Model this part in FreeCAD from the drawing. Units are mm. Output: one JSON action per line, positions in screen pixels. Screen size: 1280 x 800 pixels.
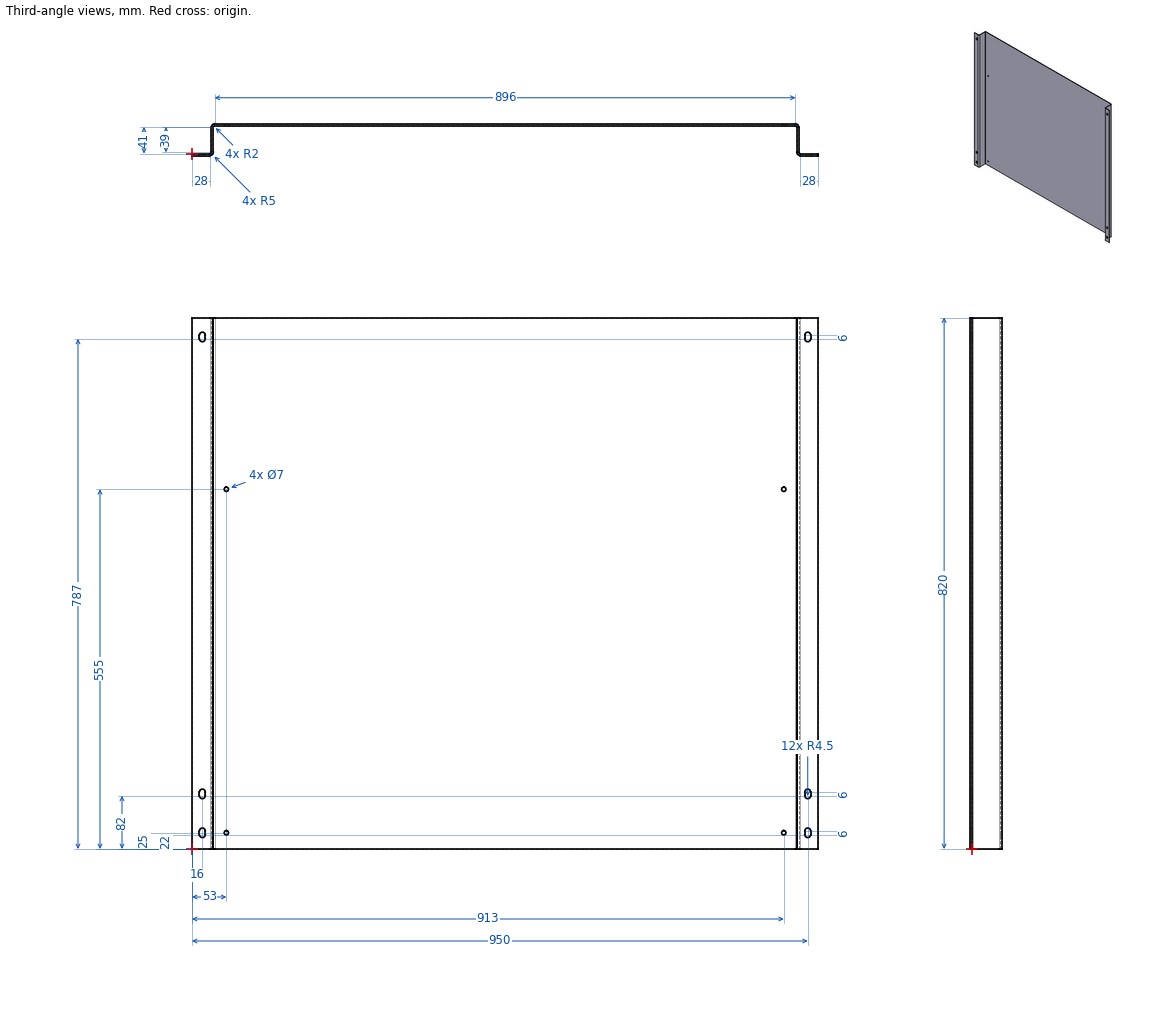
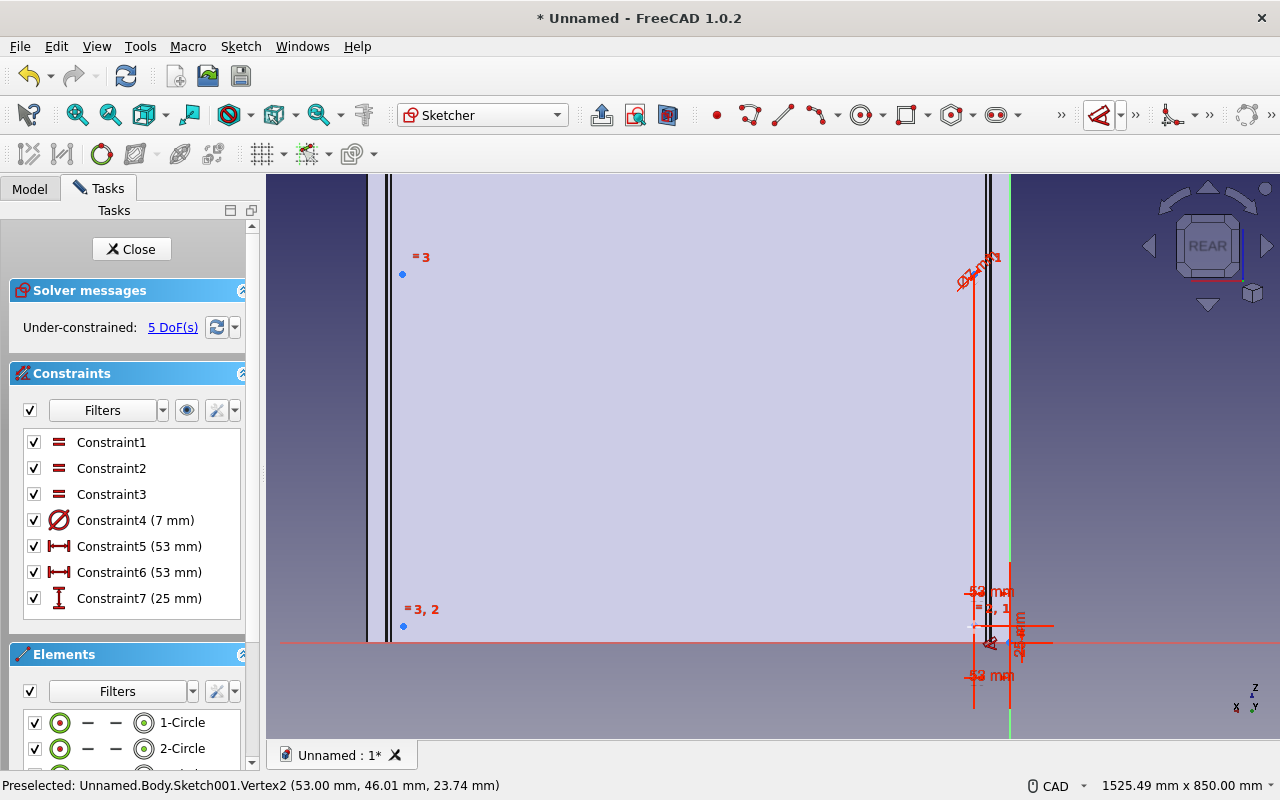
{"action": "scroll", "coordinate": [403, 627], "scroll_direction": "up", "scroll_amount": 5}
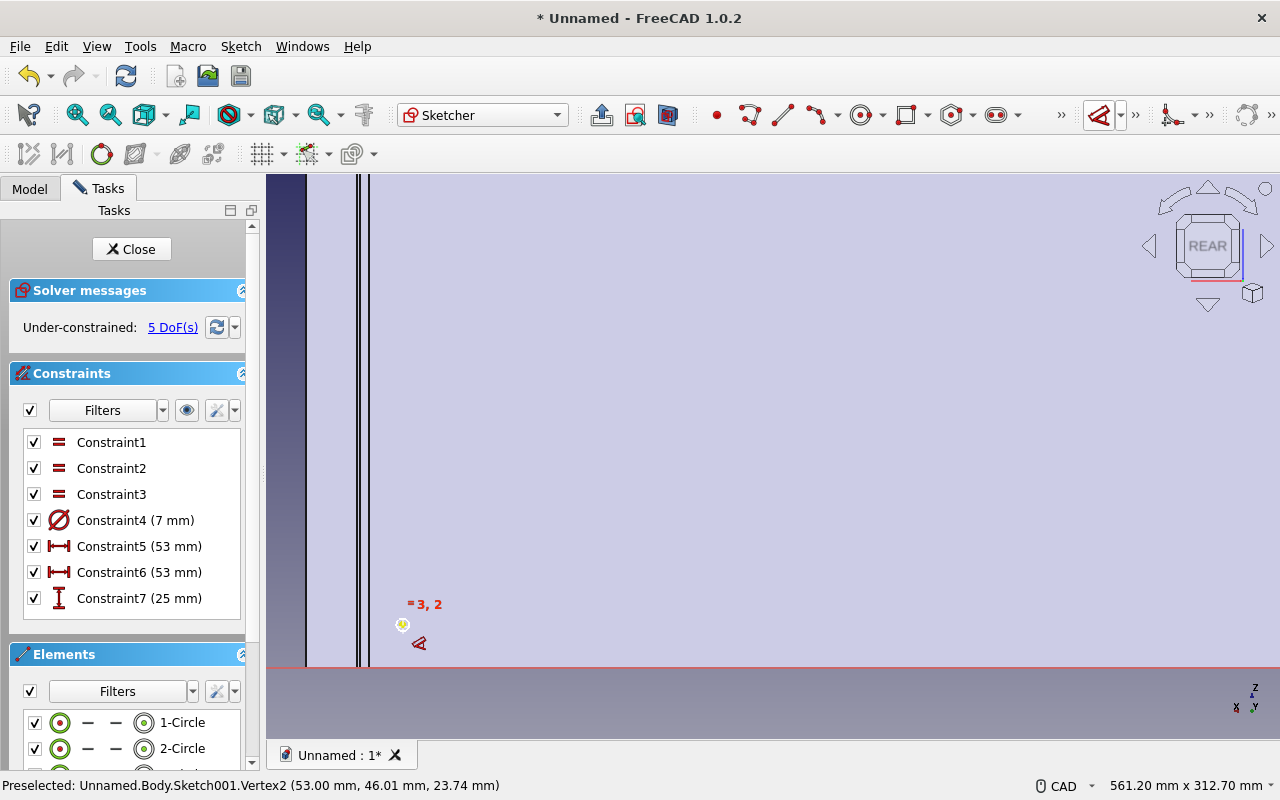
{"action": "left_click", "coordinate": [403, 625]}
{"action": "left_click", "coordinate": [369, 646]}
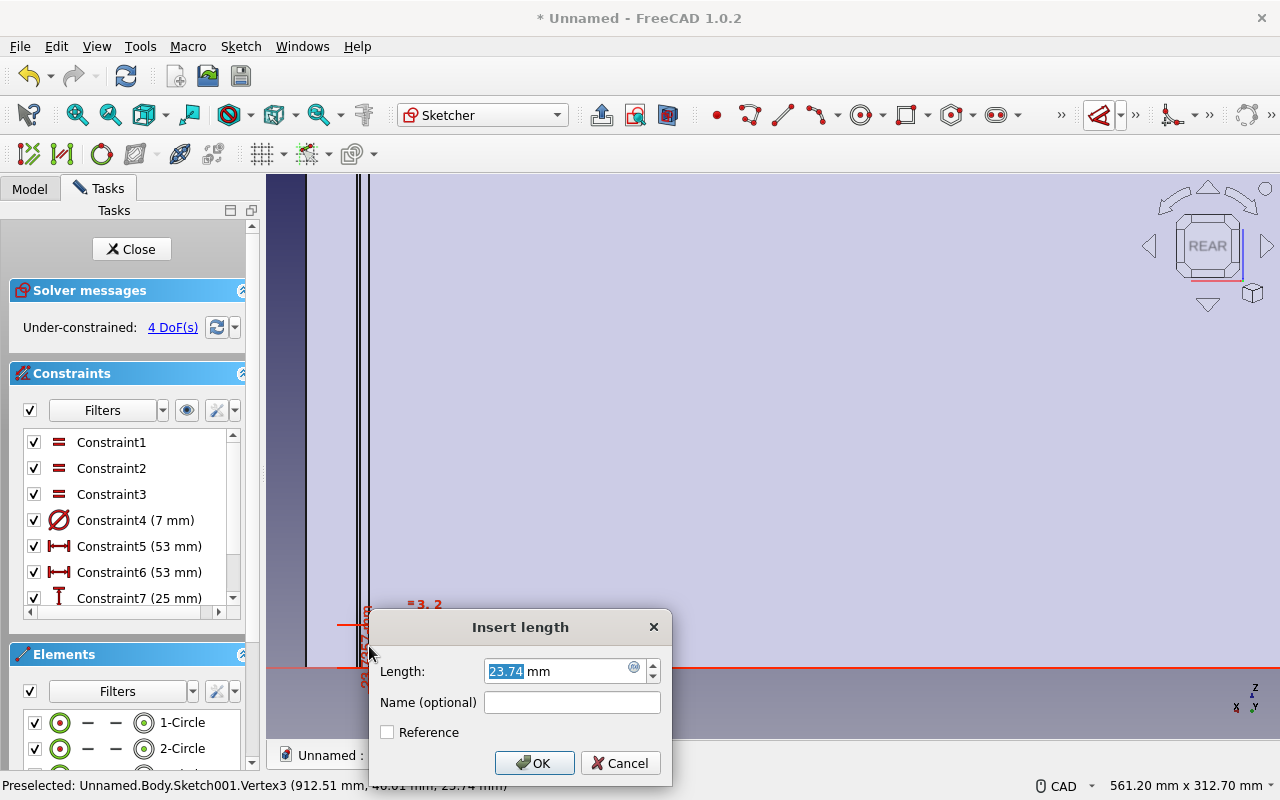
{"action": "type", "text": "25"}
{"action": "key", "text": "Return"}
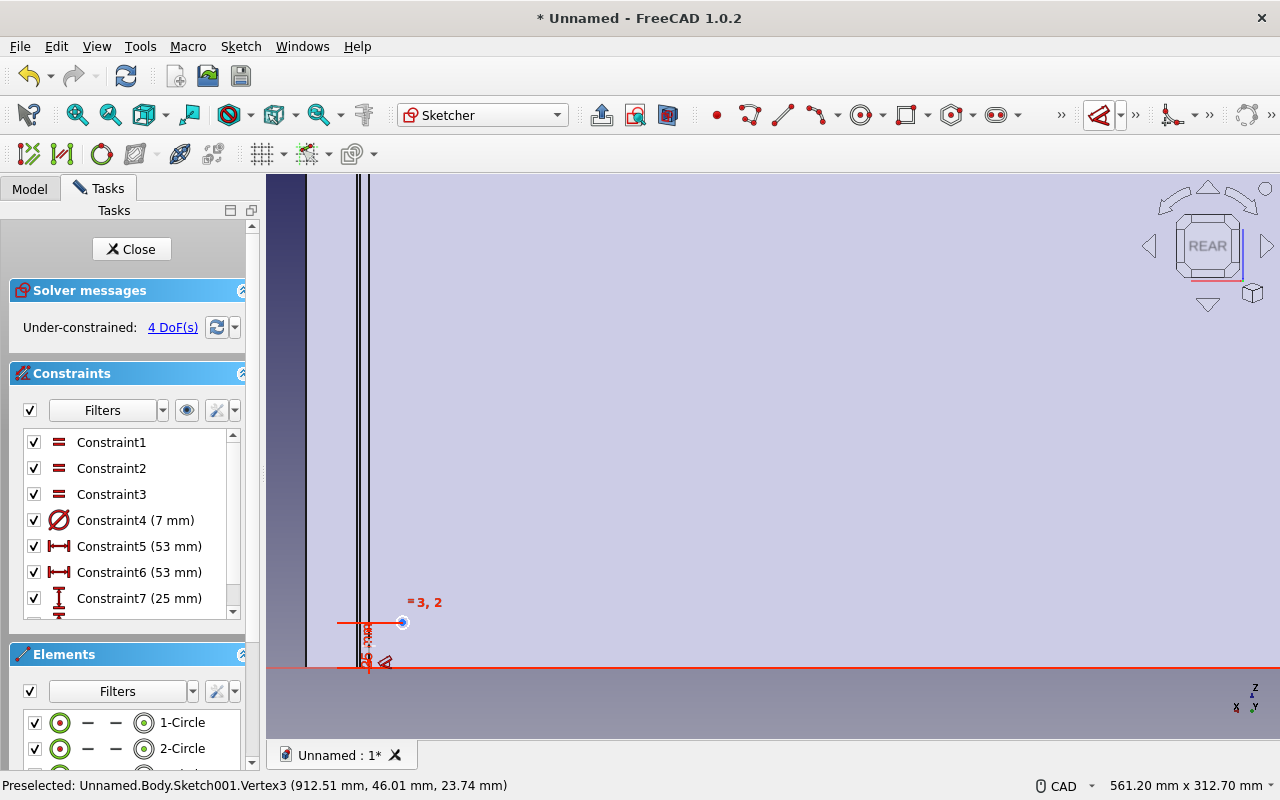
{"action": "scroll", "coordinate": [402, 627], "scroll_direction": "down", "scroll_amount": 5}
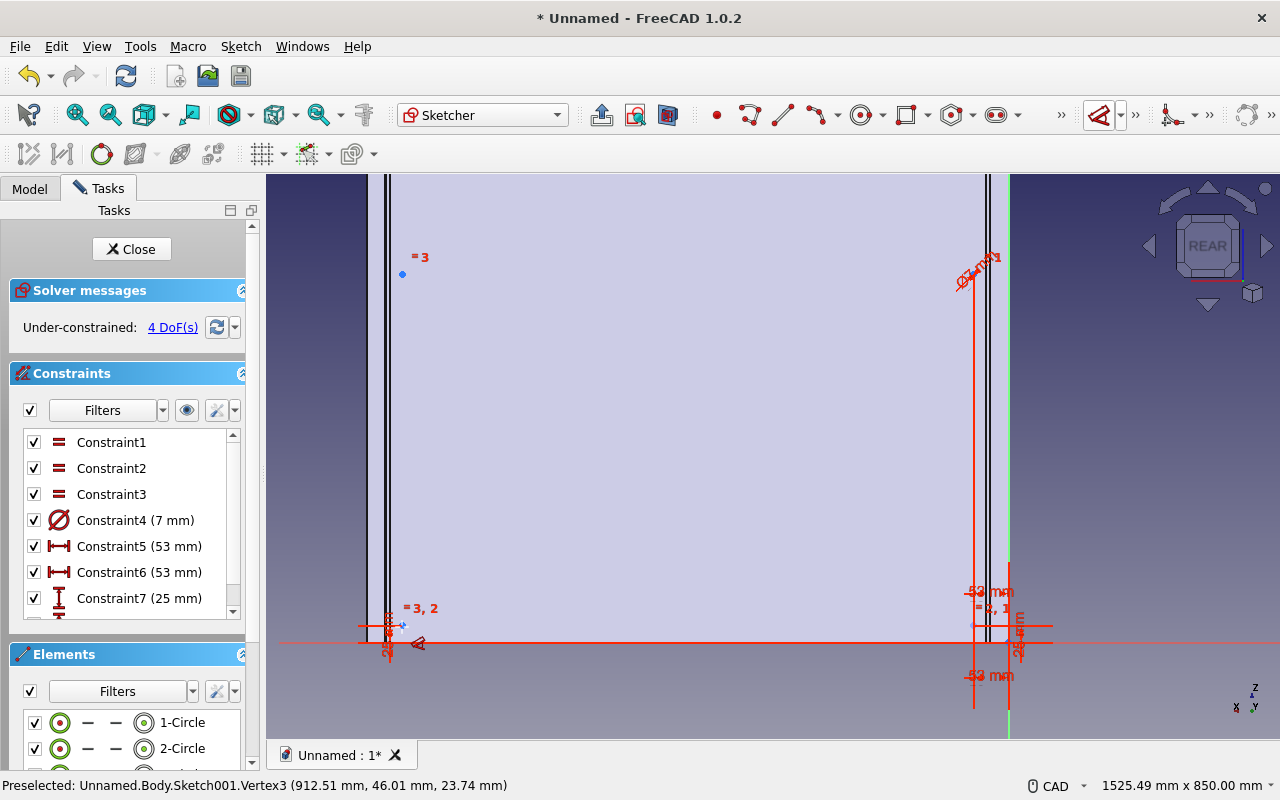
{"action": "left_click", "coordinate": [974, 275]}
{"action": "left_click", "coordinate": [1043, 459]}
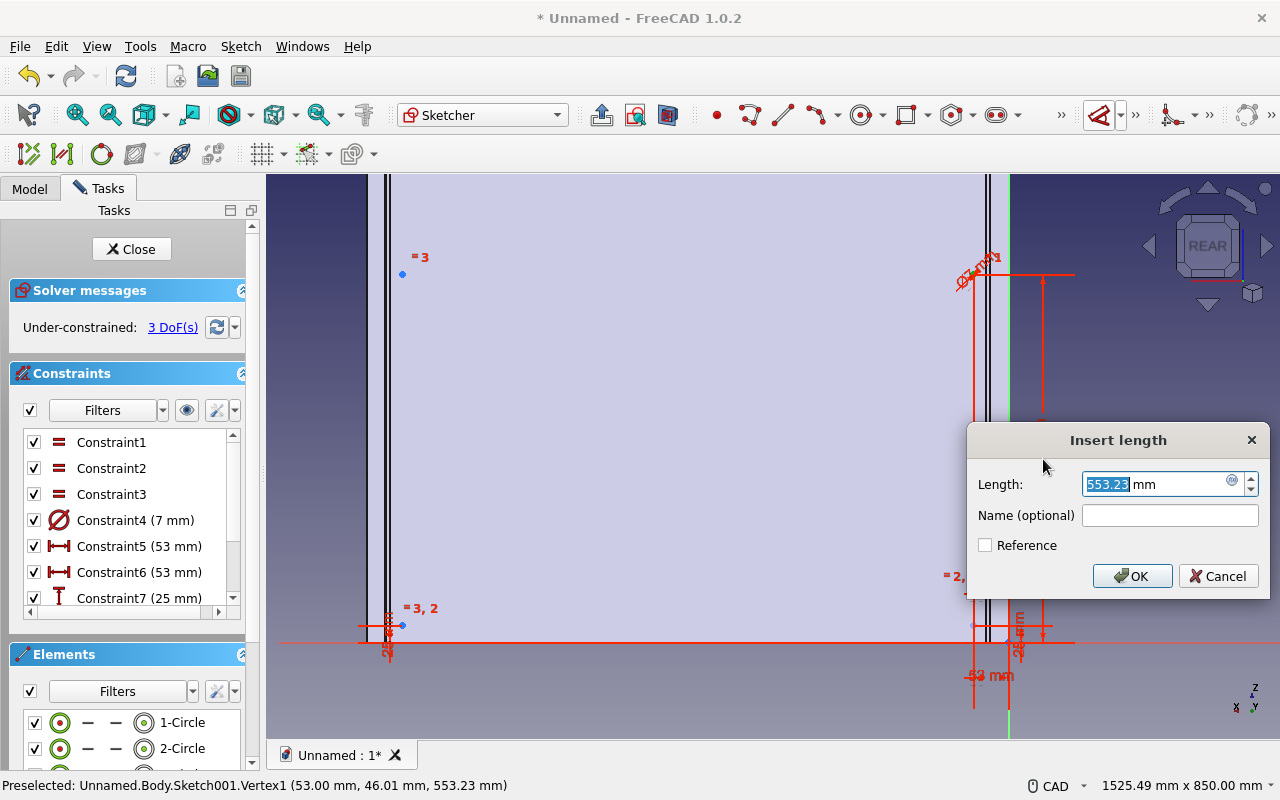
{"action": "type", "text": "555"}
{"action": "key", "text": "Return"}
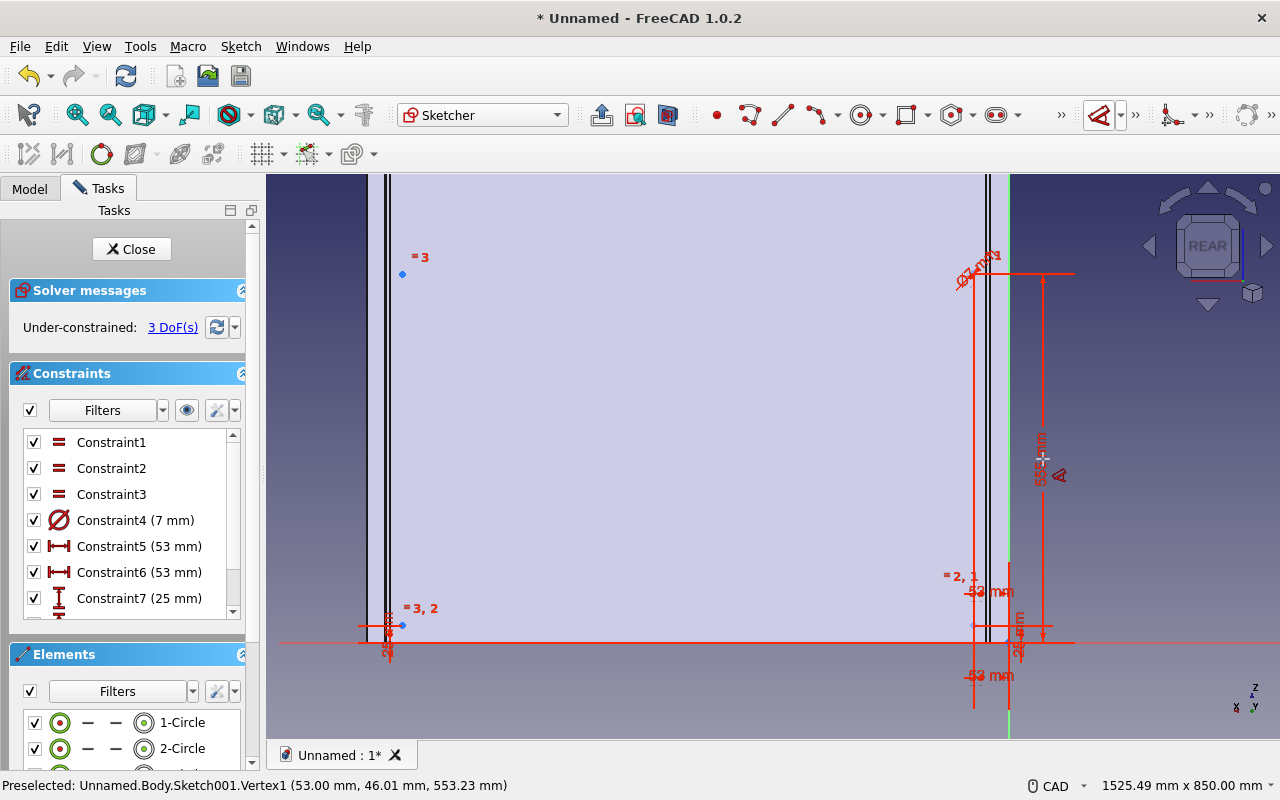
{"action": "left_click", "coordinate": [402, 626]}
{"action": "left_click", "coordinate": [706, 676]}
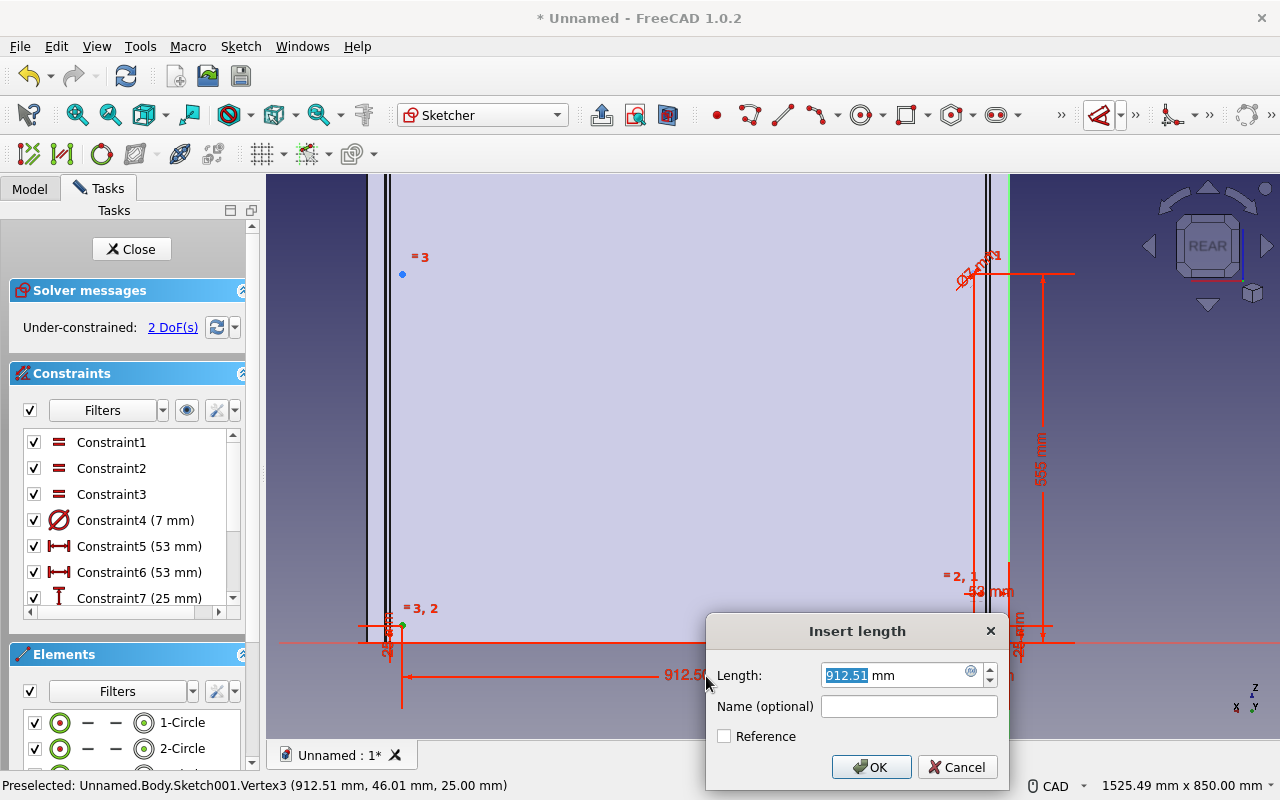
{"action": "type", "text": "913"}
{"action": "key", "text": "Return"}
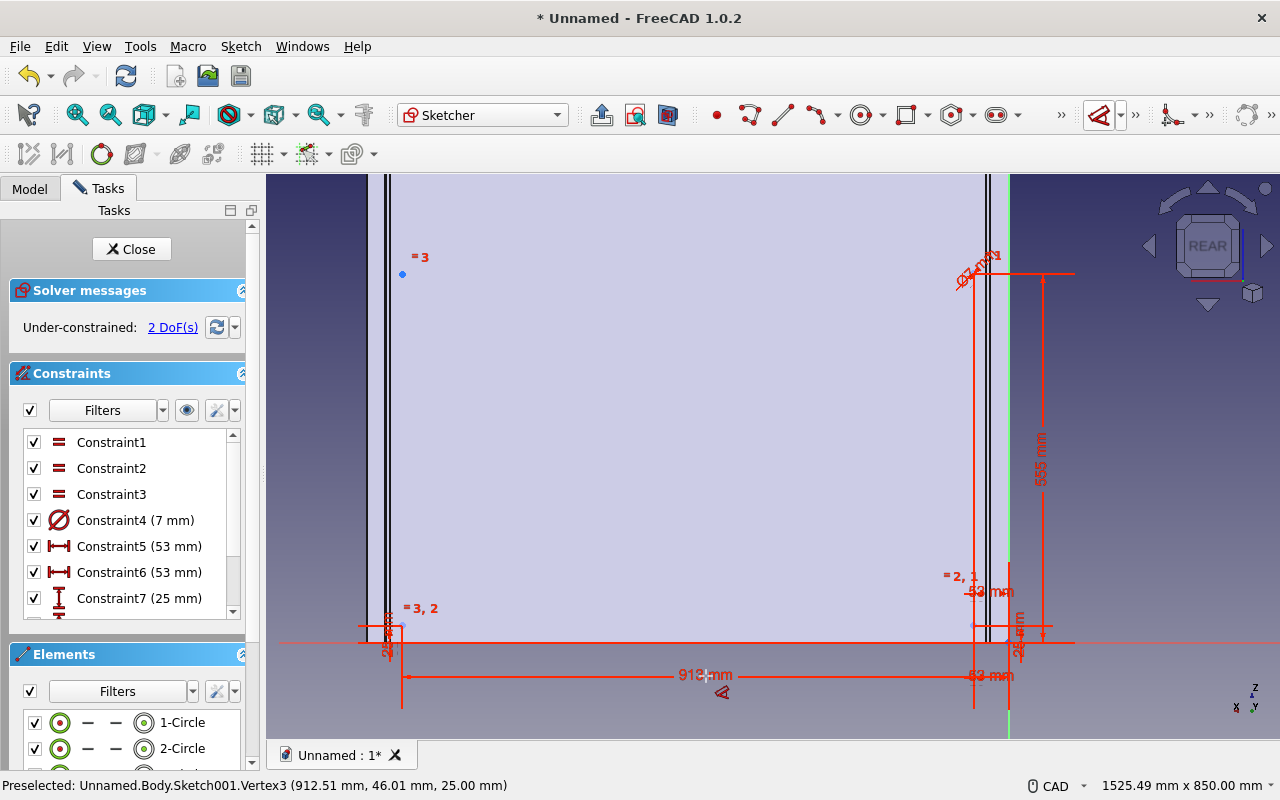
{"action": "left_click", "coordinate": [402, 275]}
{"action": "left_click", "coordinate": [566, 676]}